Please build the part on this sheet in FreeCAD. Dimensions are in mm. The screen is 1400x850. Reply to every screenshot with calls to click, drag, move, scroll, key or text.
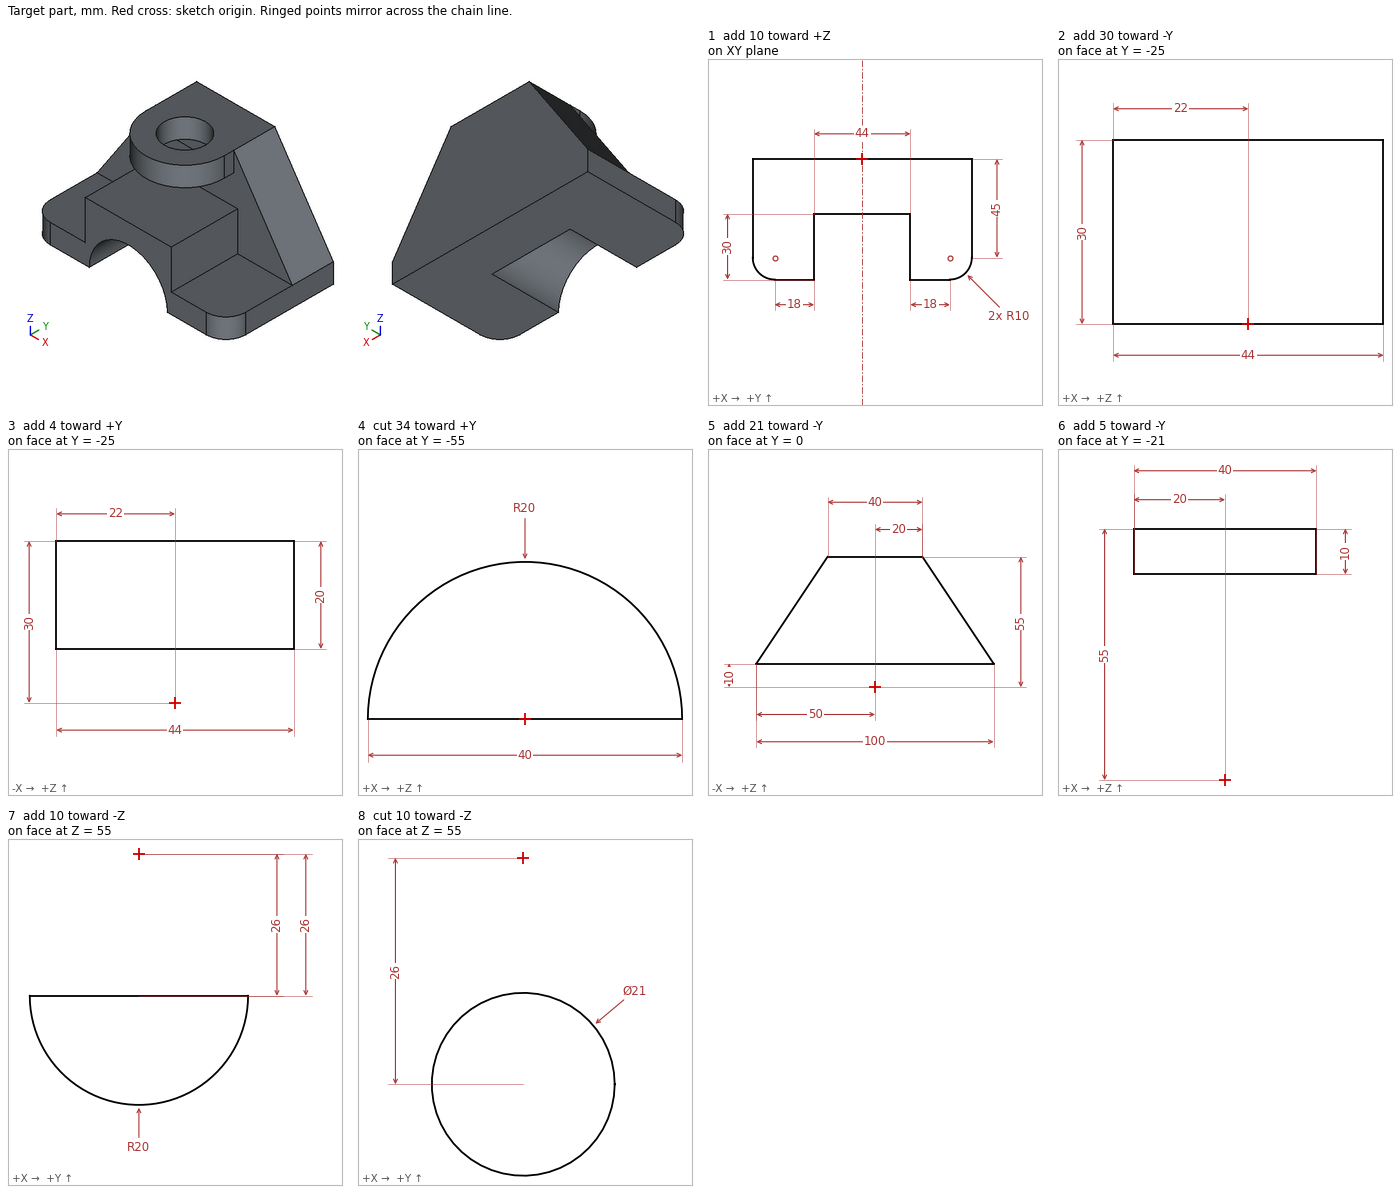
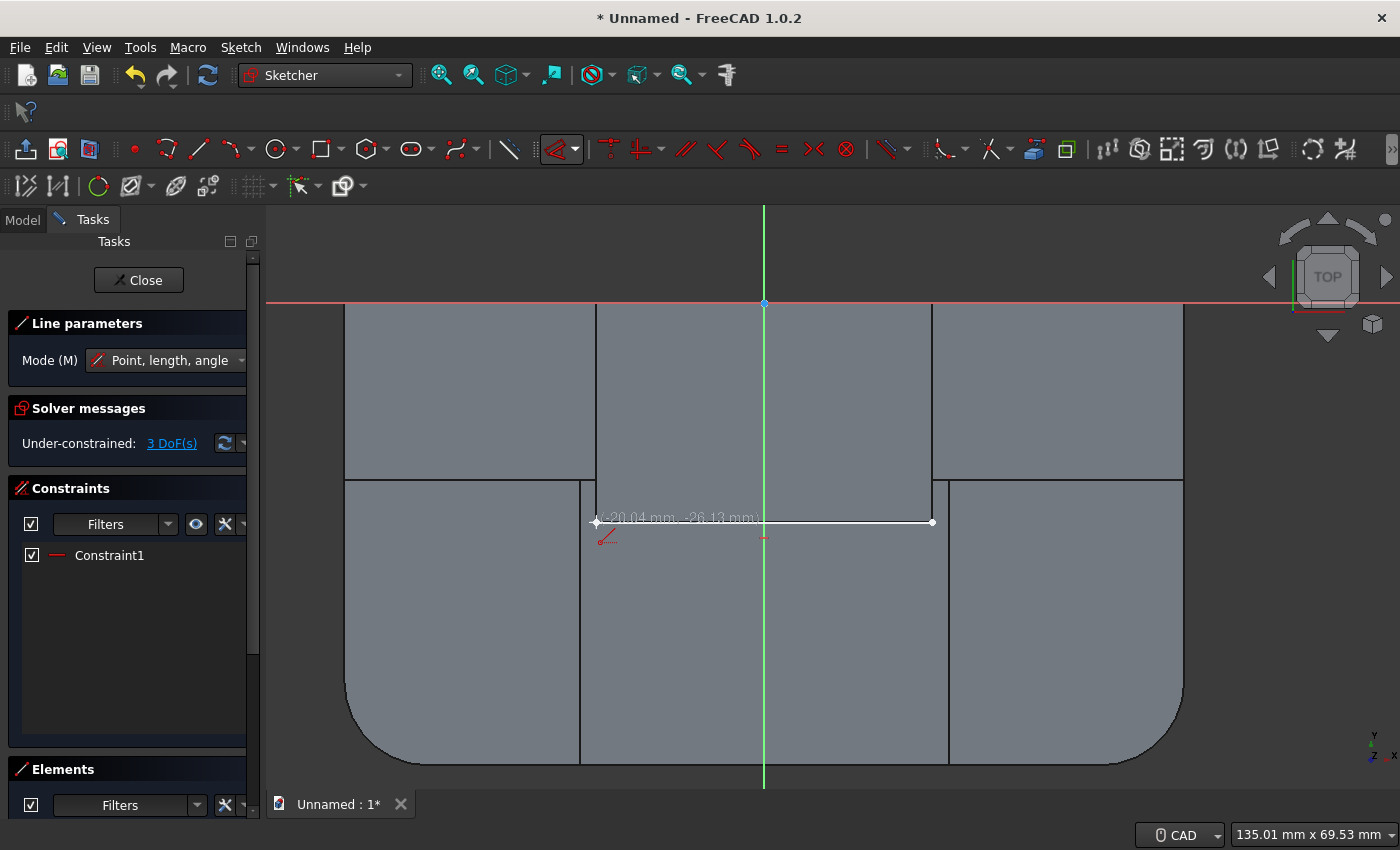
click(232, 150)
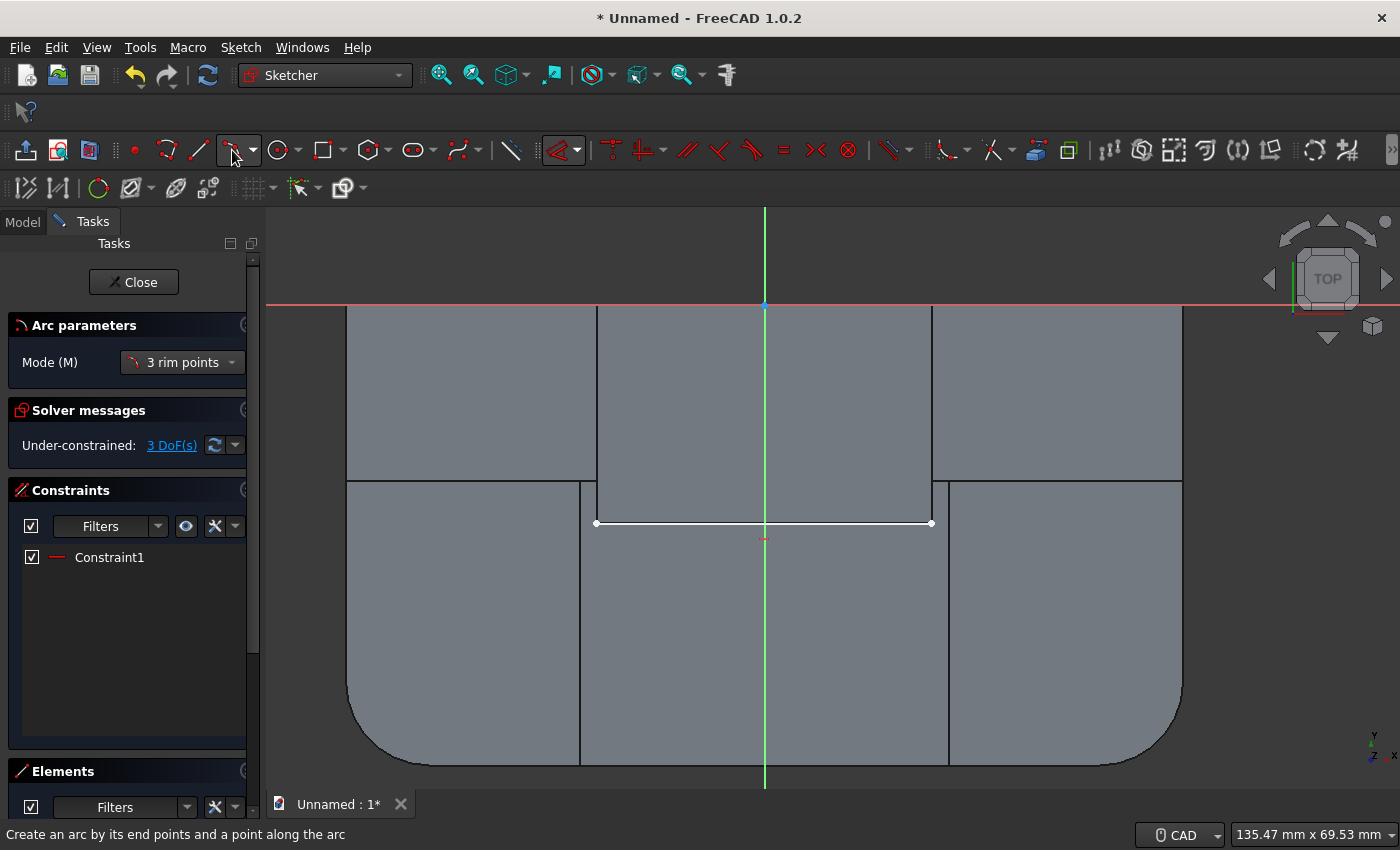
click(597, 524)
click(932, 524)
click(713, 682)
key(Escape)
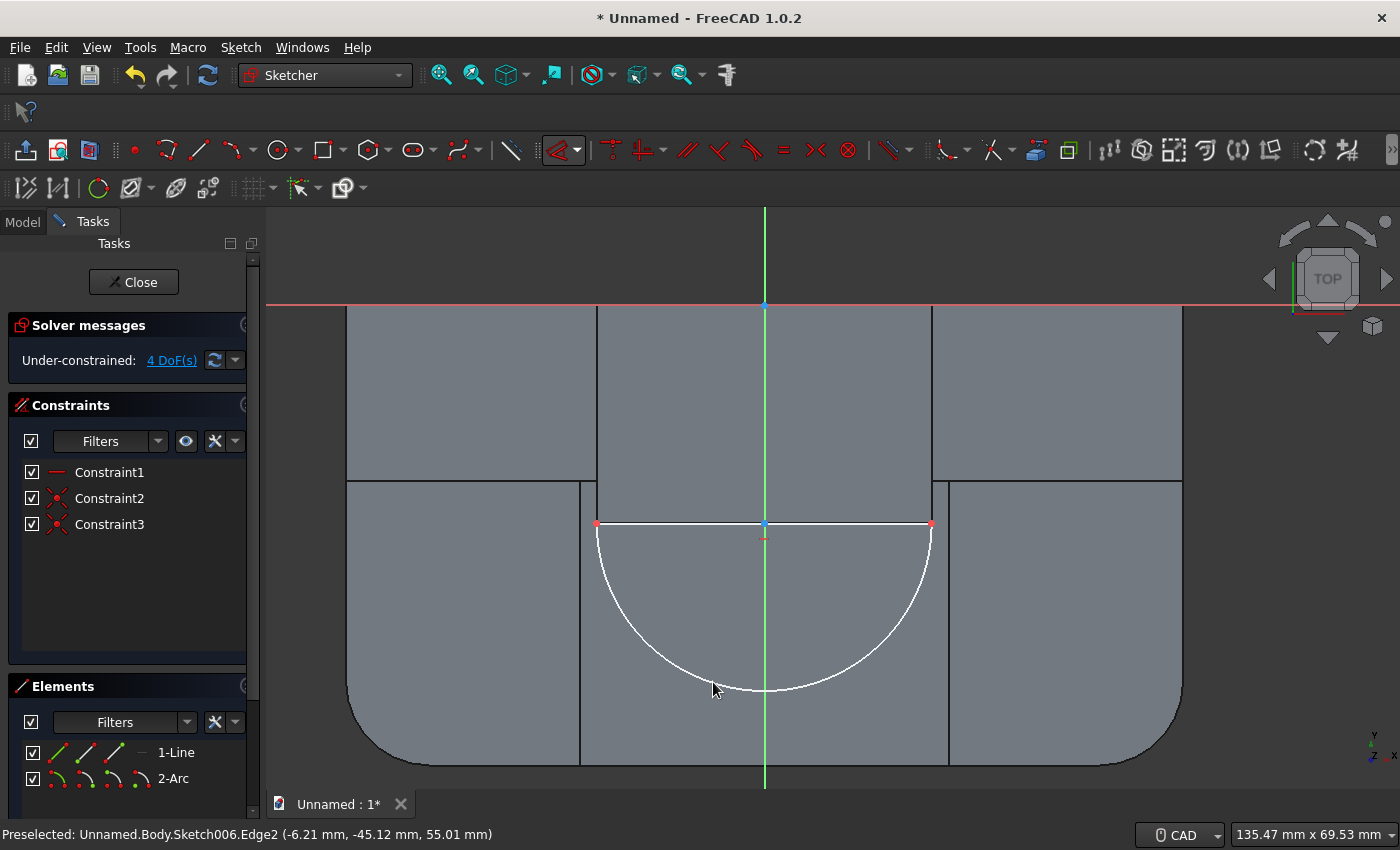
click(764, 524)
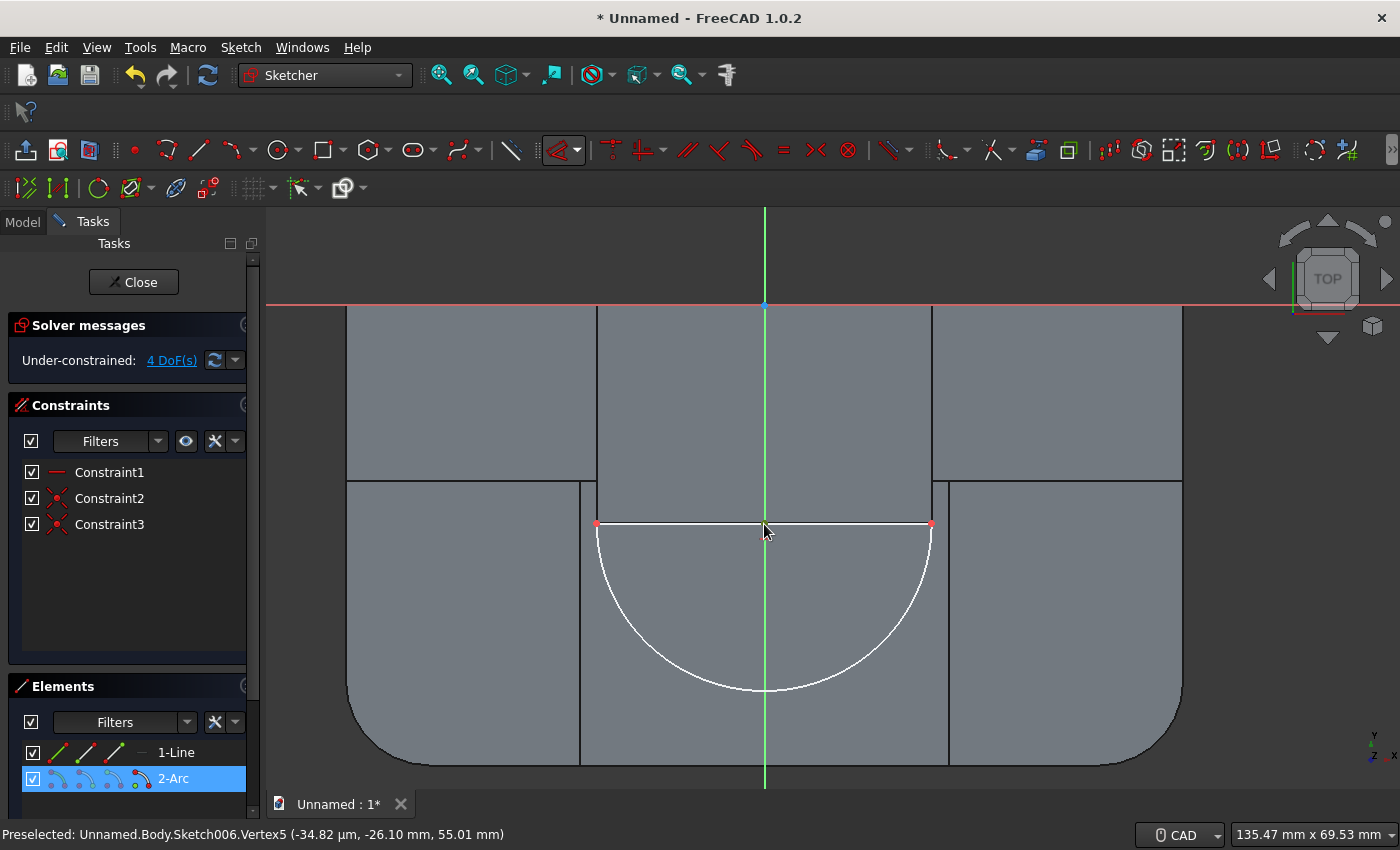
click(765, 723)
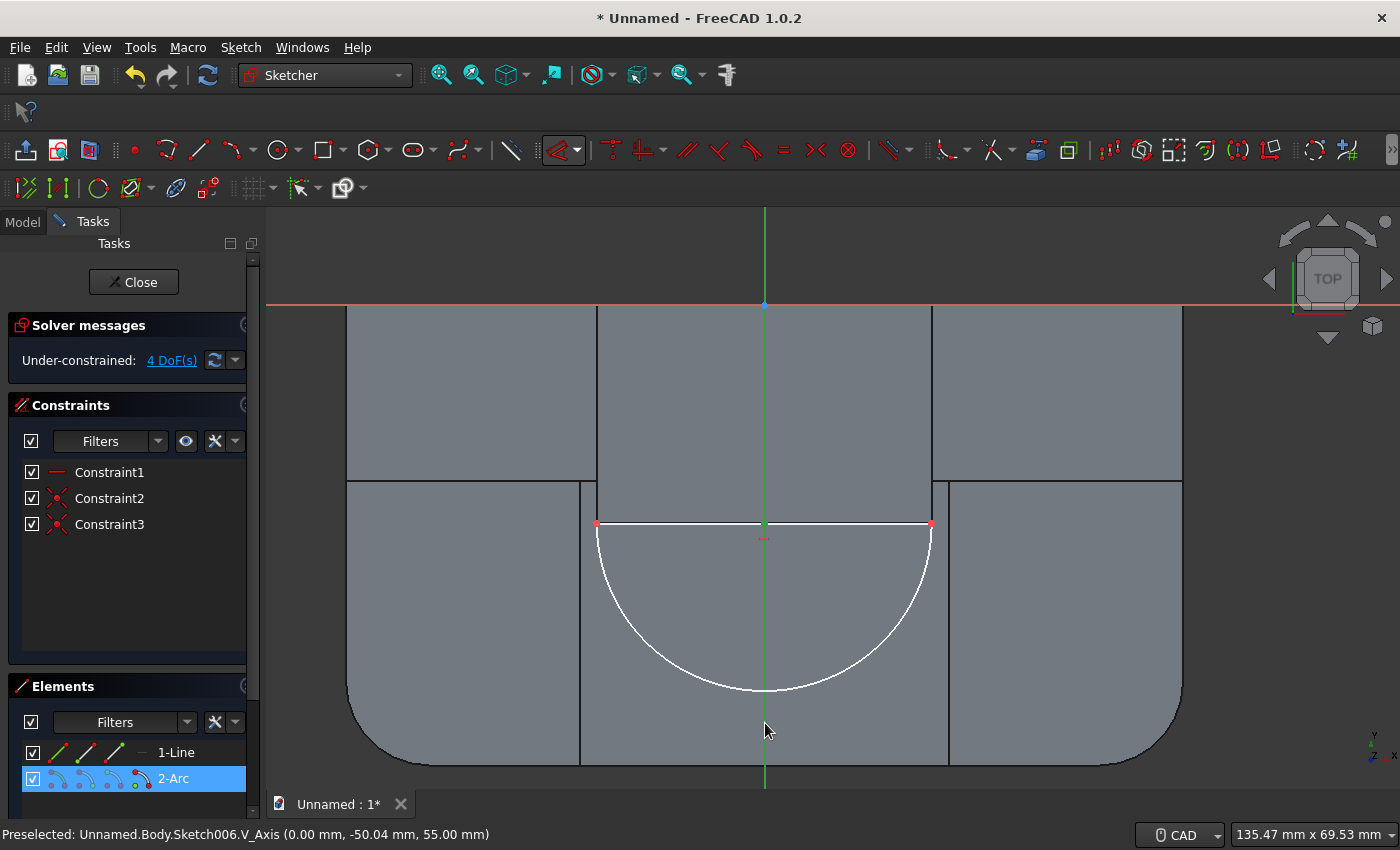
click(612, 150)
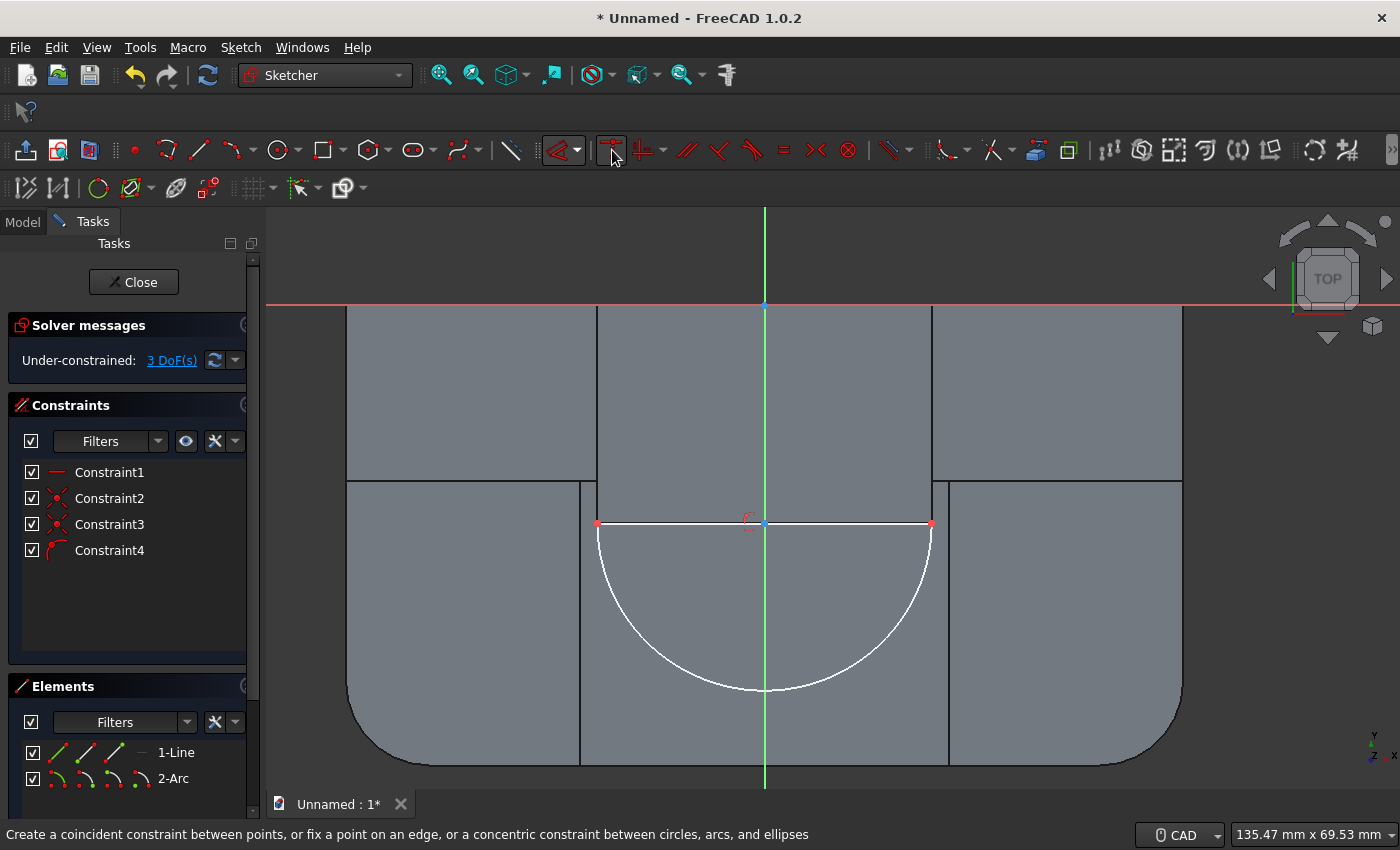
click(666, 659)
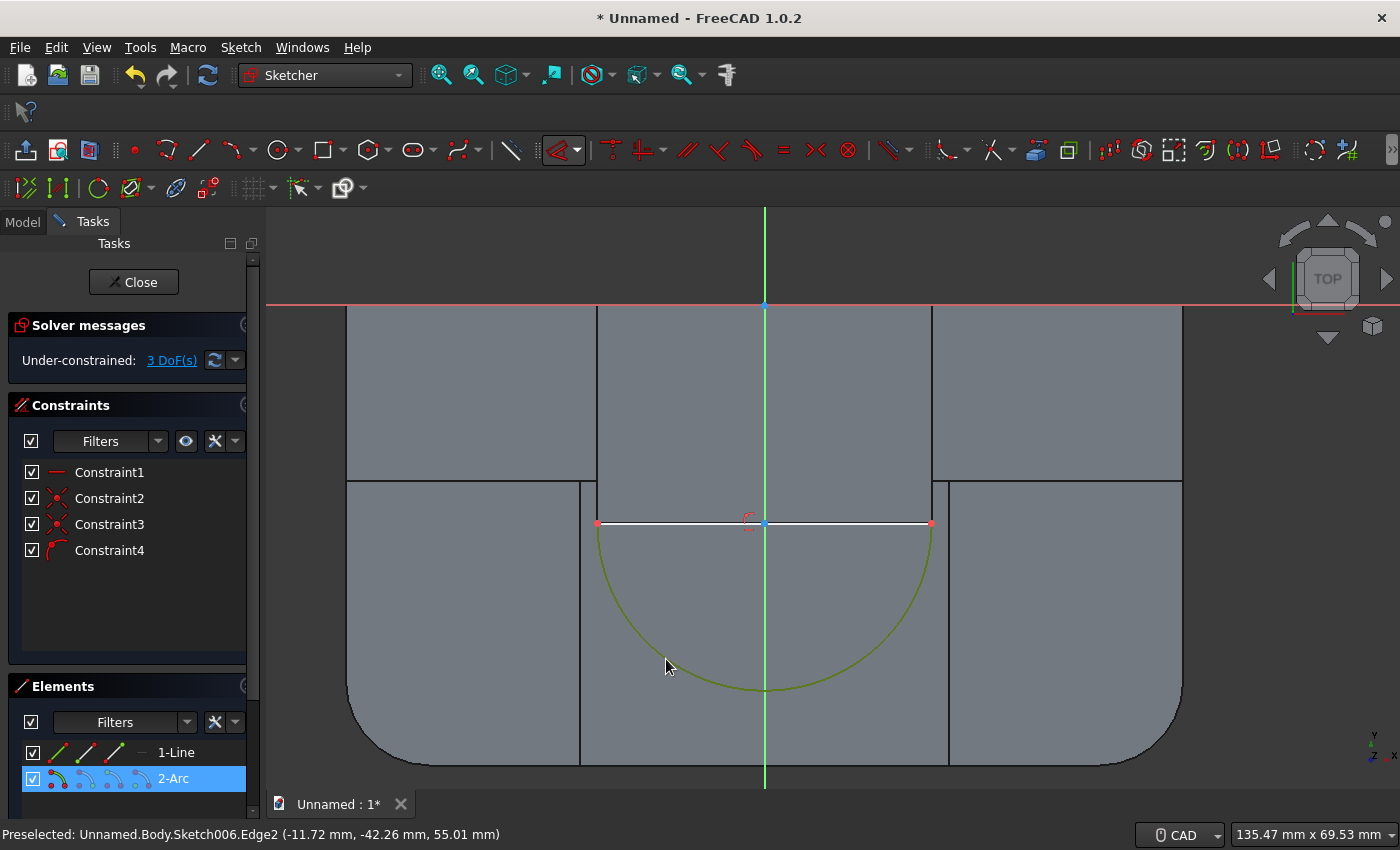
key(k)
key(r)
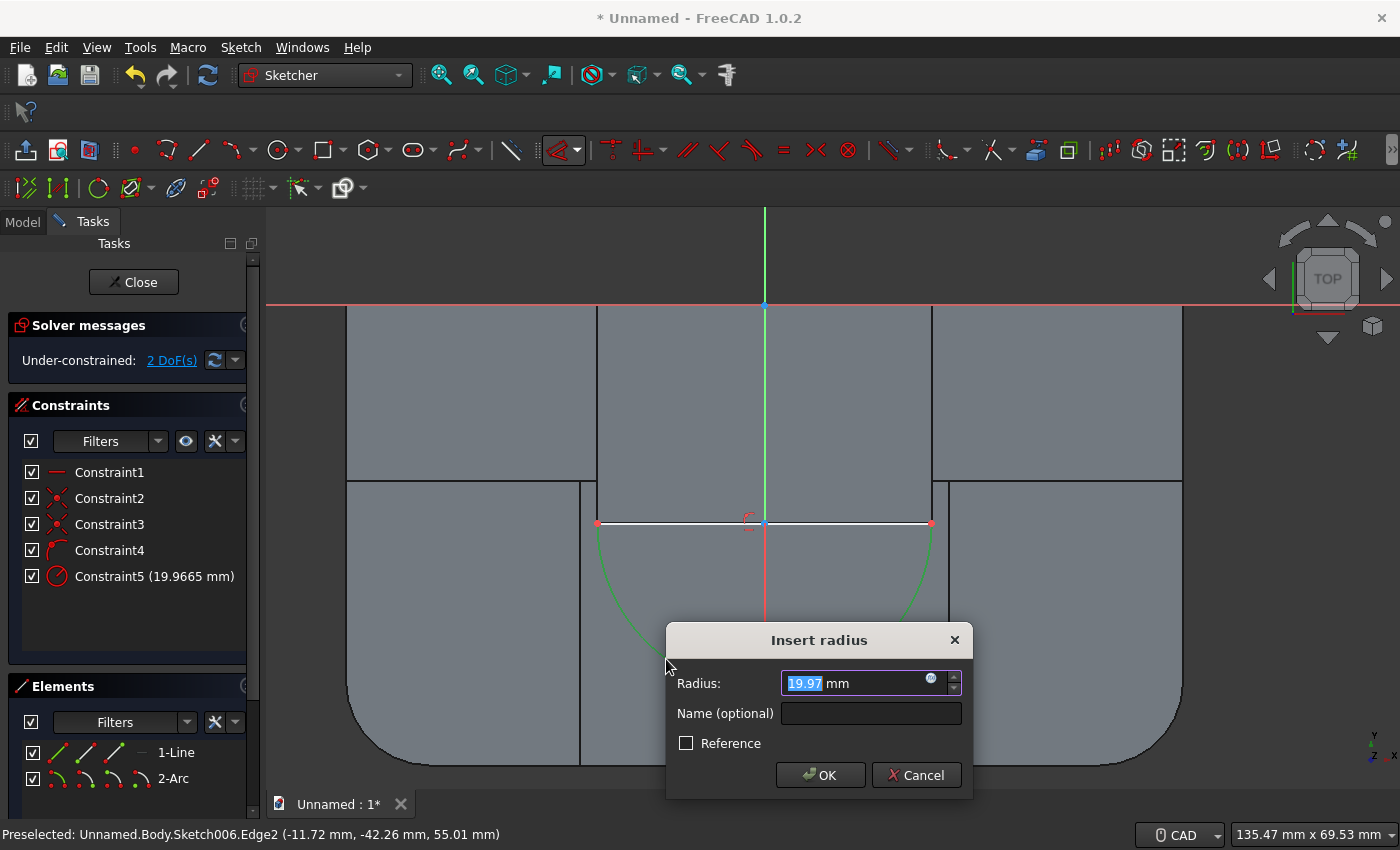
text(20)
key(Return)